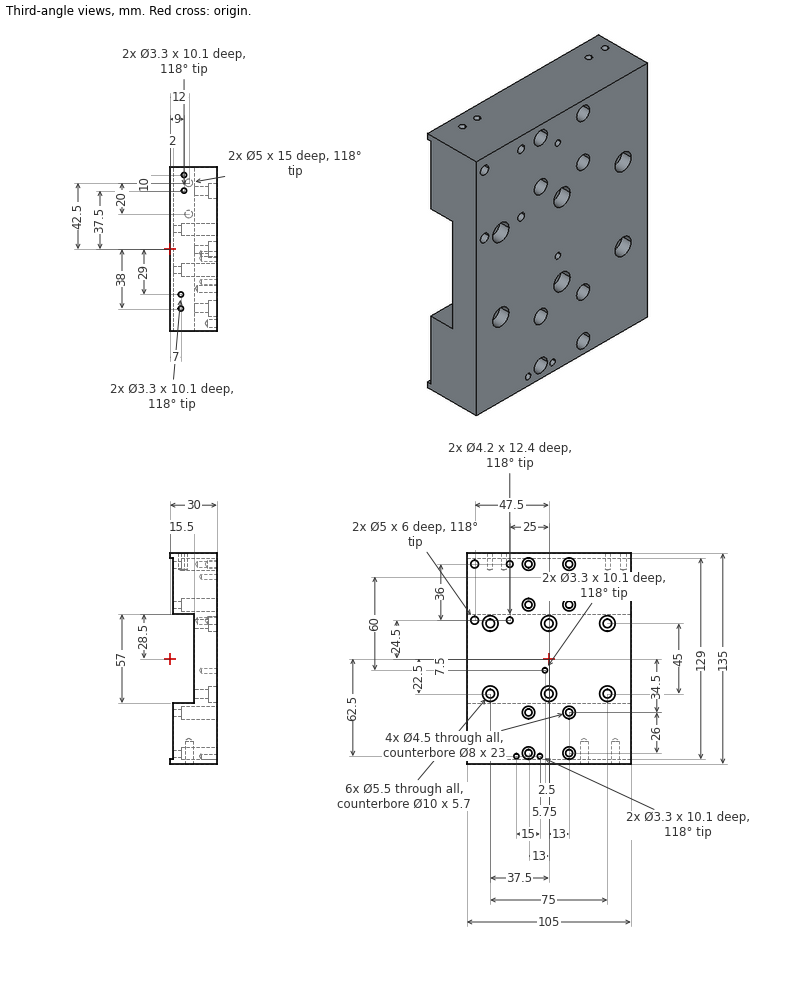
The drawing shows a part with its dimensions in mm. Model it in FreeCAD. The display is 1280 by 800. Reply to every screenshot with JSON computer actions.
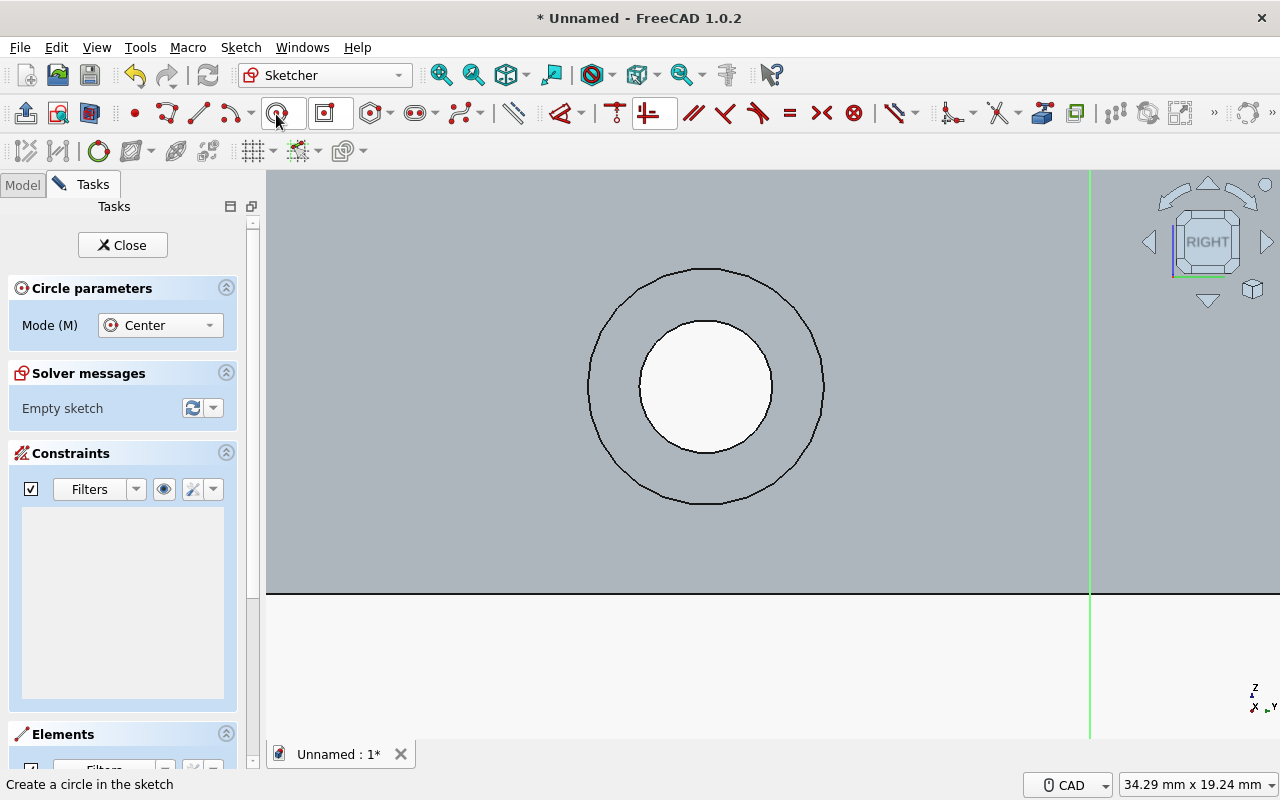
{"action": "left_click", "coordinate": [920, 446]}
{"action": "left_click", "coordinate": [955, 411]}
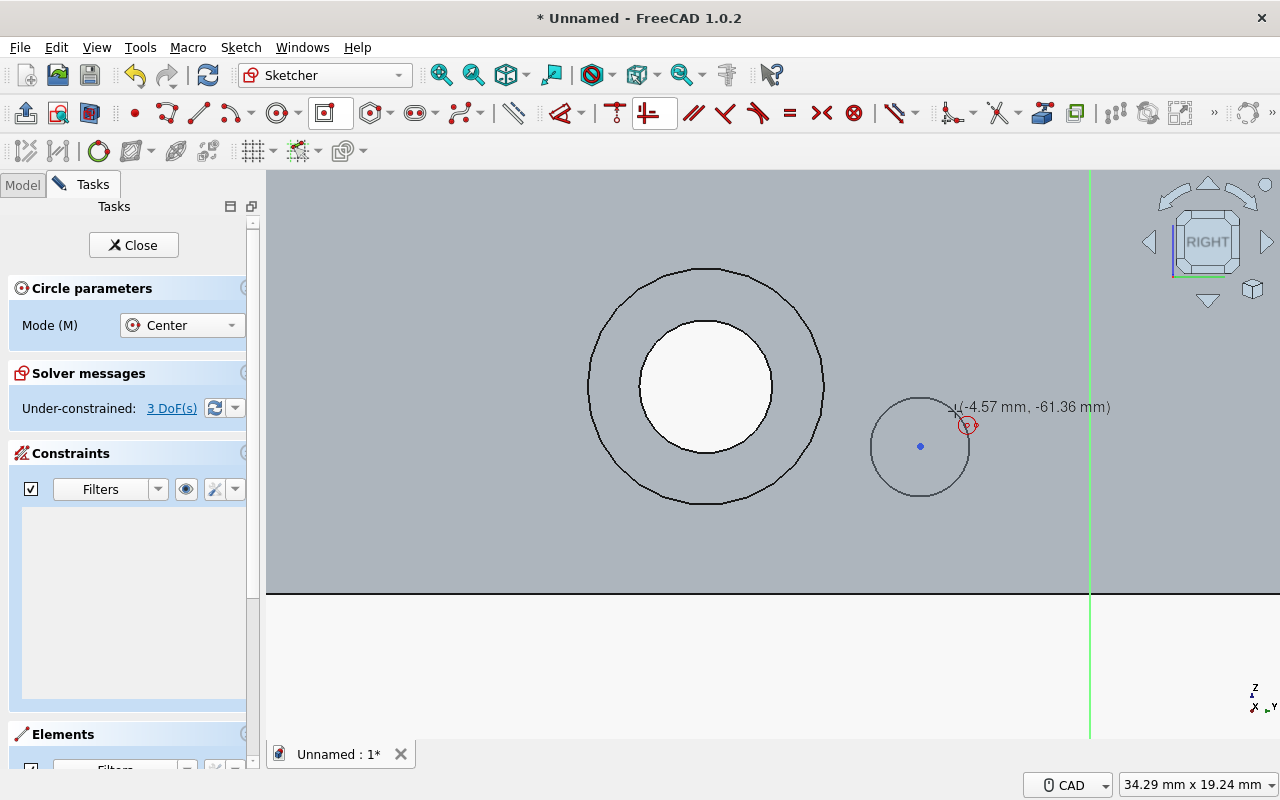
{"action": "left_click", "coordinate": [477, 446]}
{"action": "left_click", "coordinate": [511, 411]}
{"action": "key", "text": "Escape"}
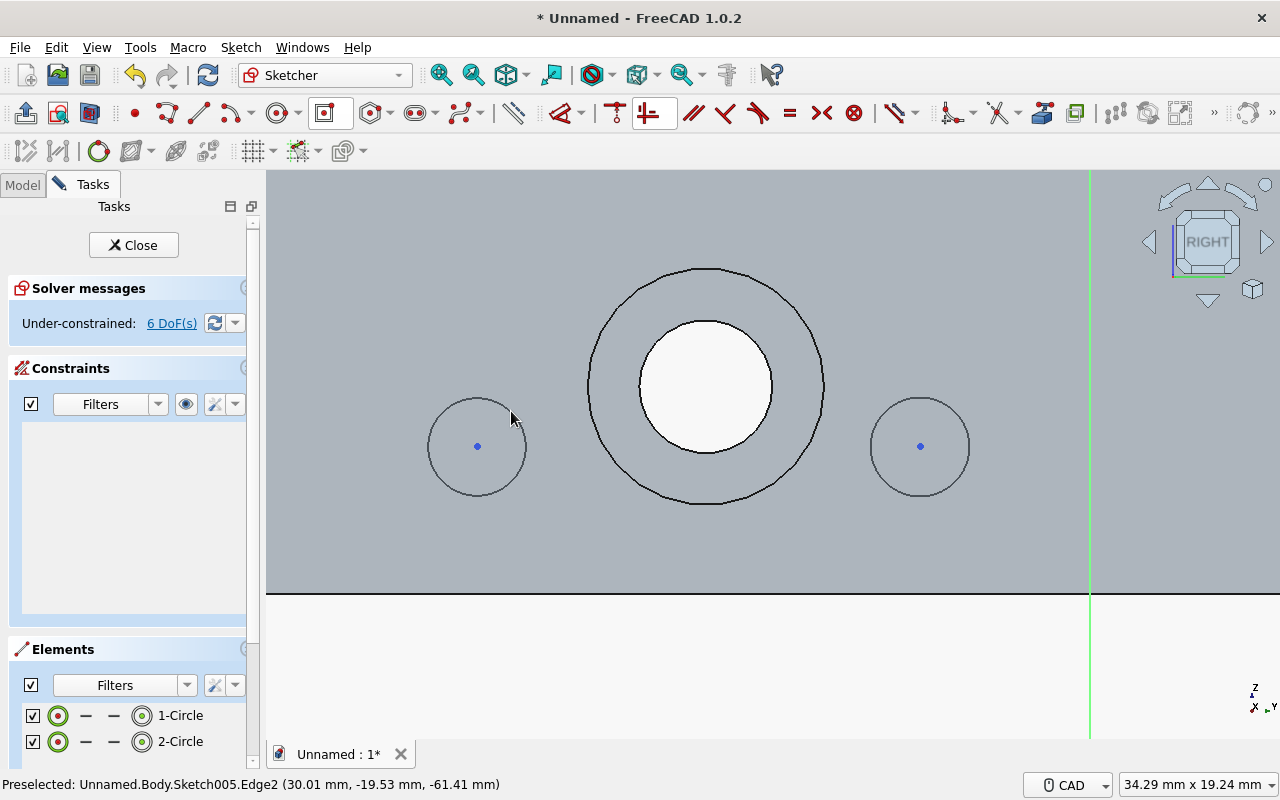
{"action": "left_click", "coordinate": [955, 412]}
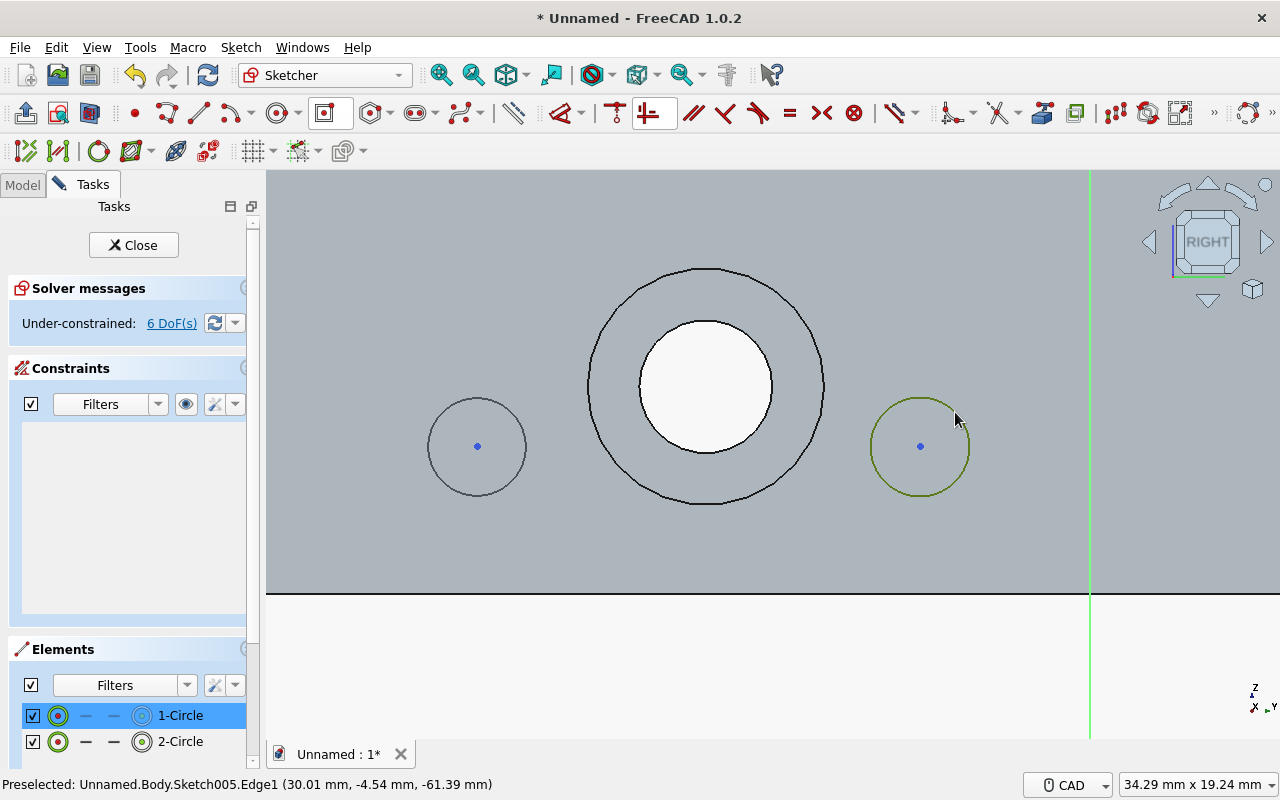
{"action": "left_click", "coordinate": [511, 412]}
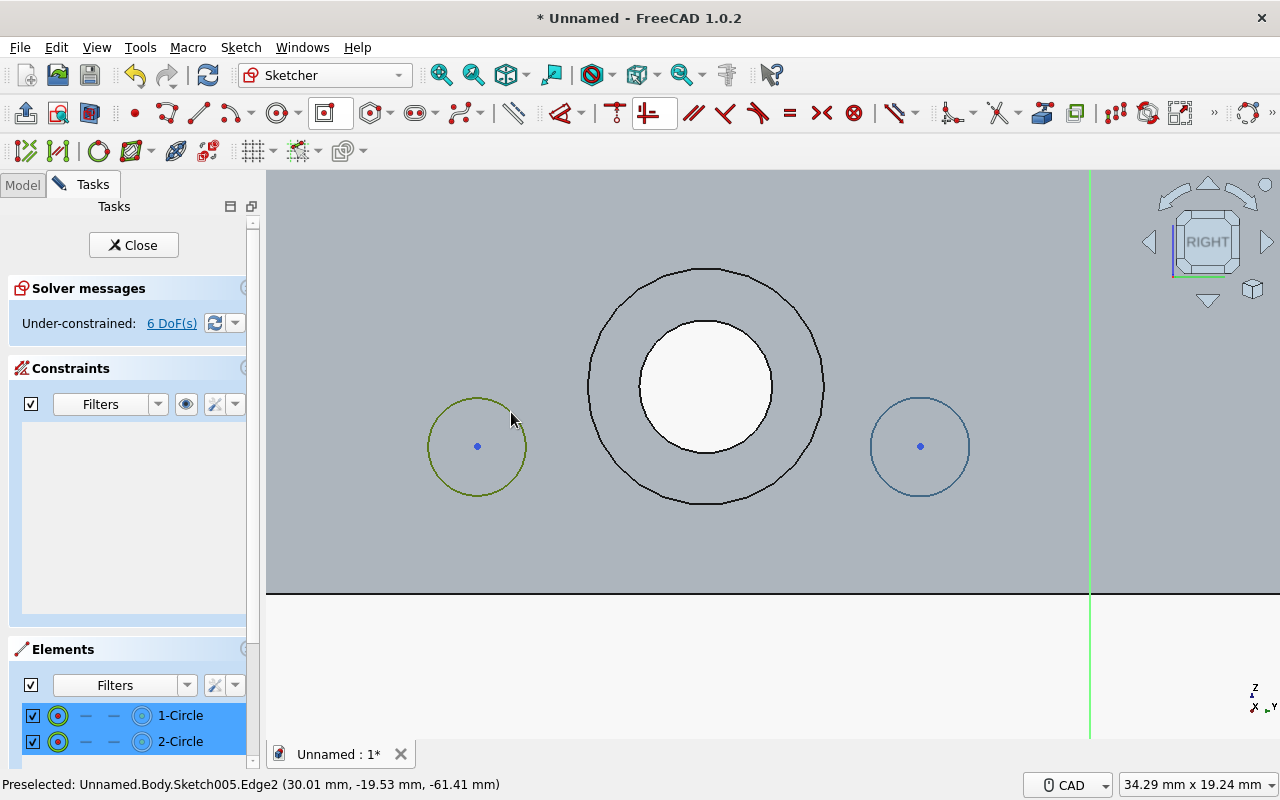
{"action": "left_click", "coordinate": [790, 114]}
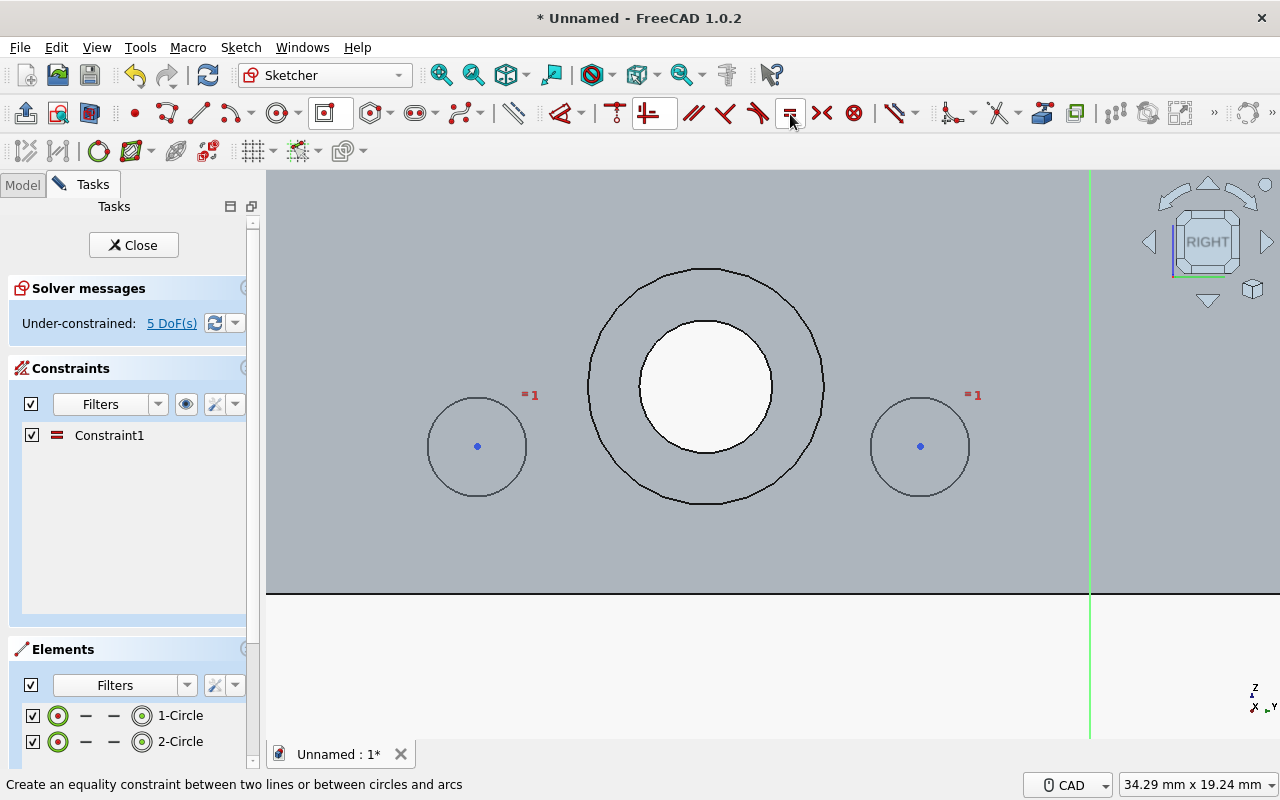
{"action": "left_click", "coordinate": [920, 447]}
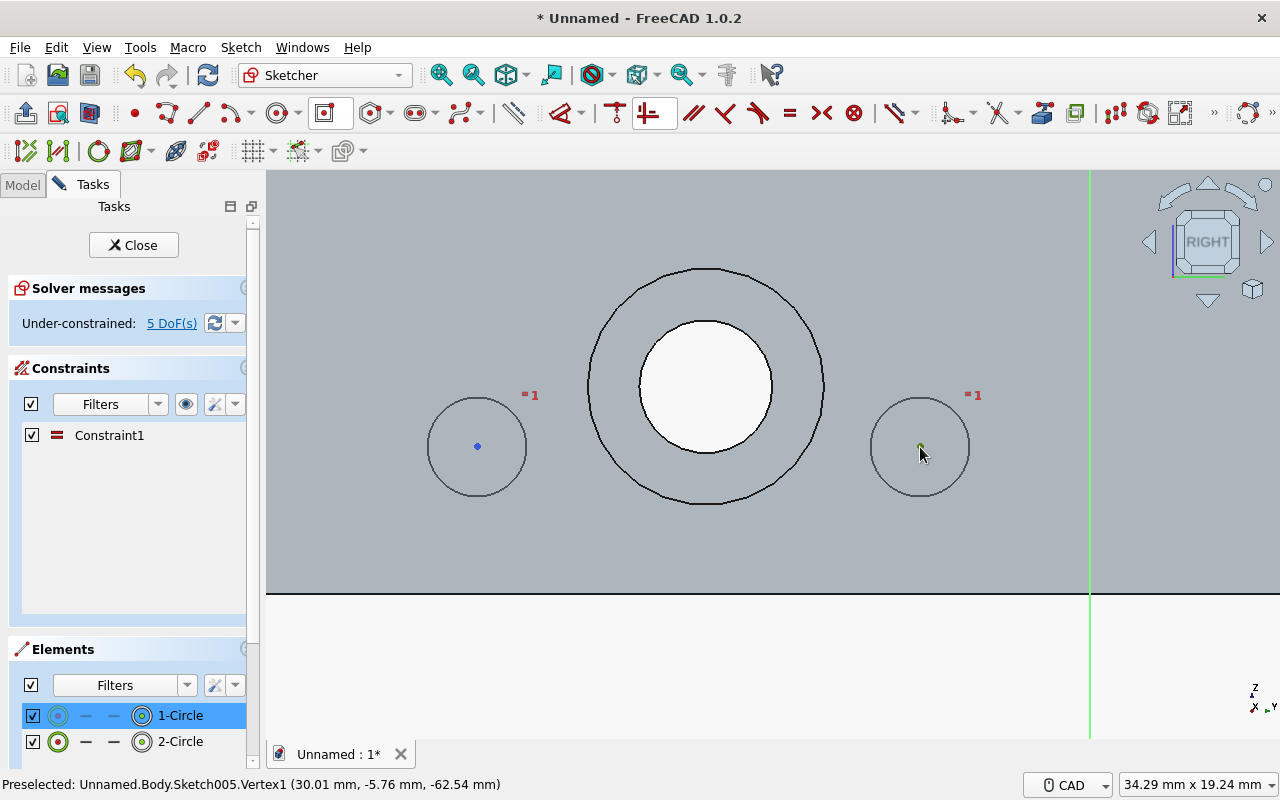
{"action": "left_click", "coordinate": [477, 447]}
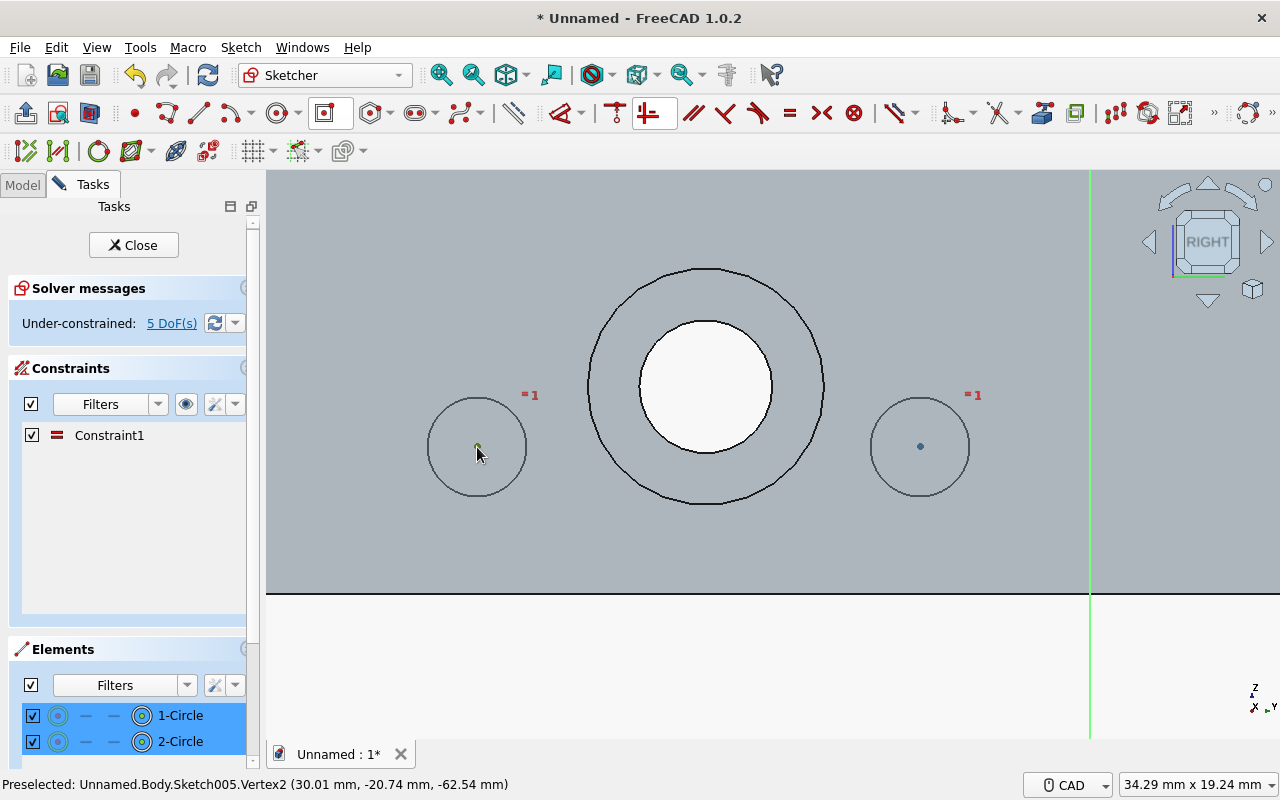
{"action": "key", "text": "h"}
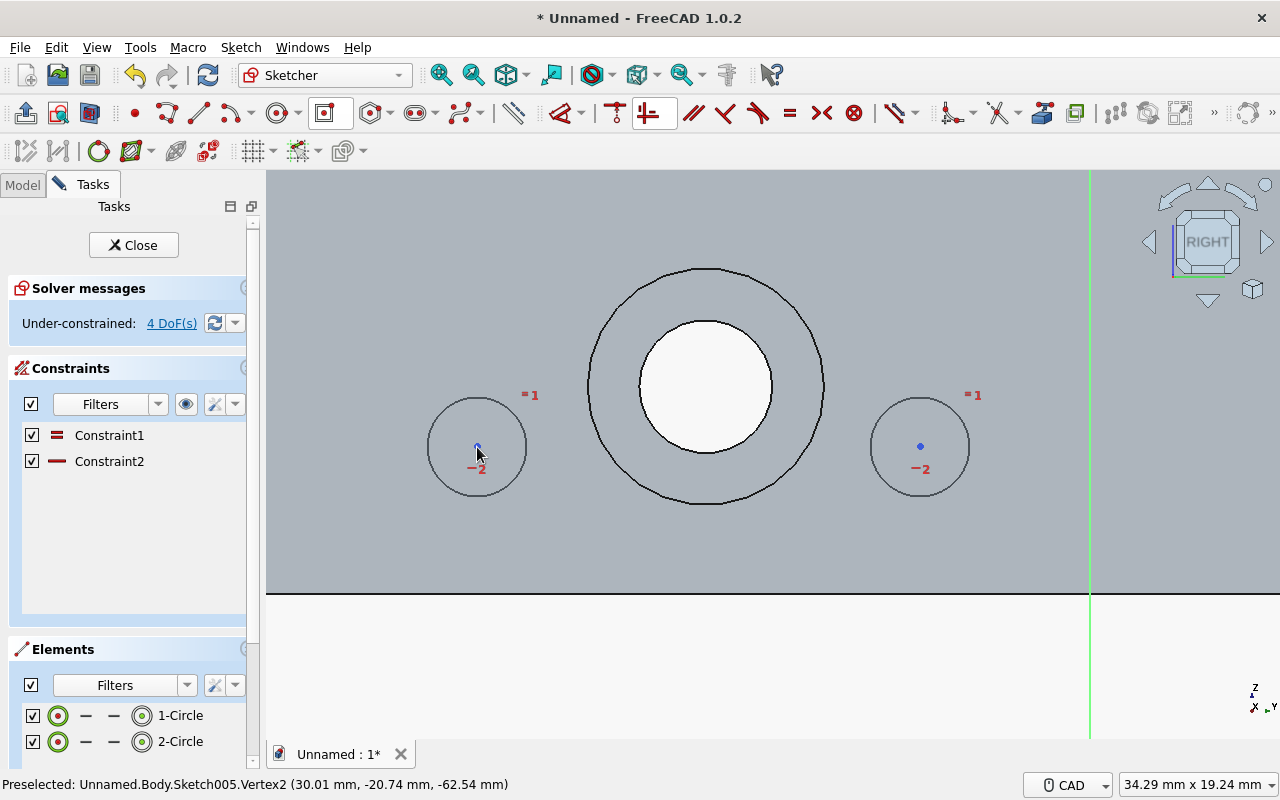
{"action": "left_click", "coordinate": [560, 114]}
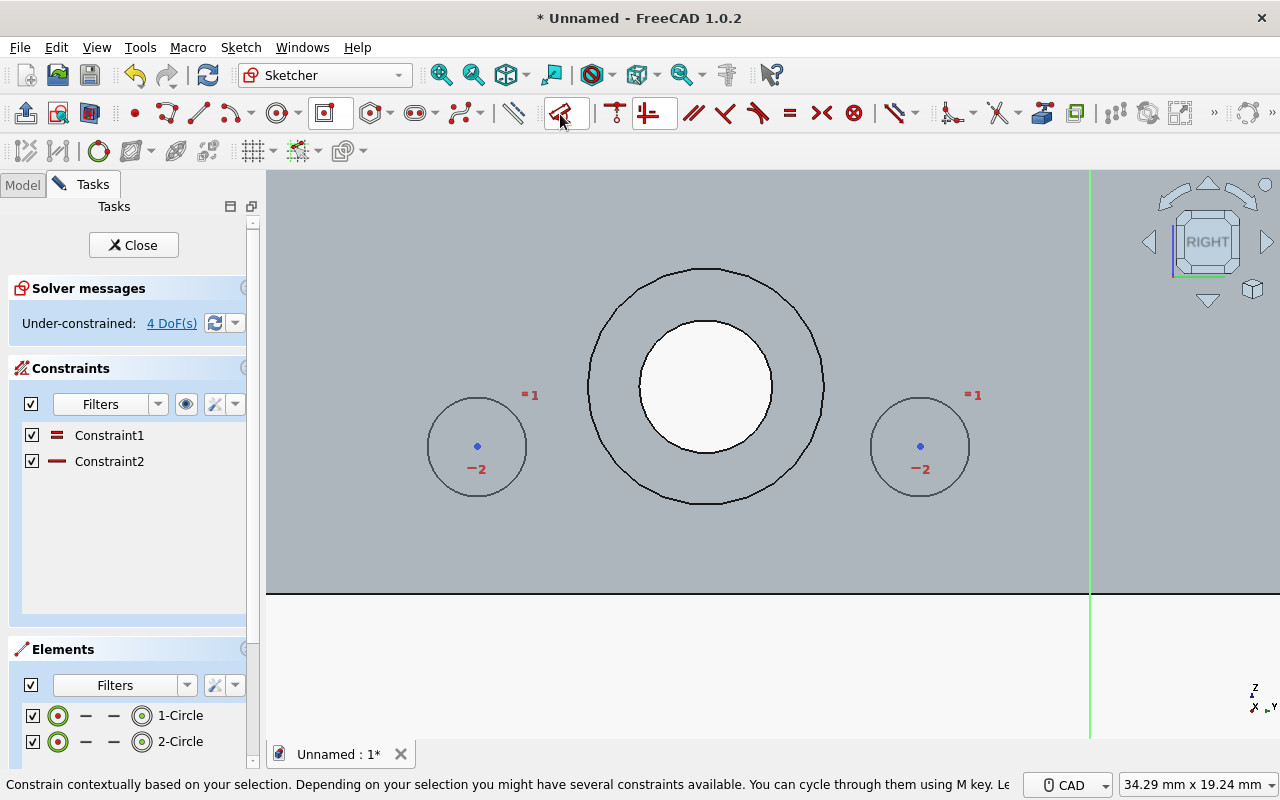
{"action": "left_click", "coordinate": [955, 412]}
{"action": "left_click", "coordinate": [978, 389]}